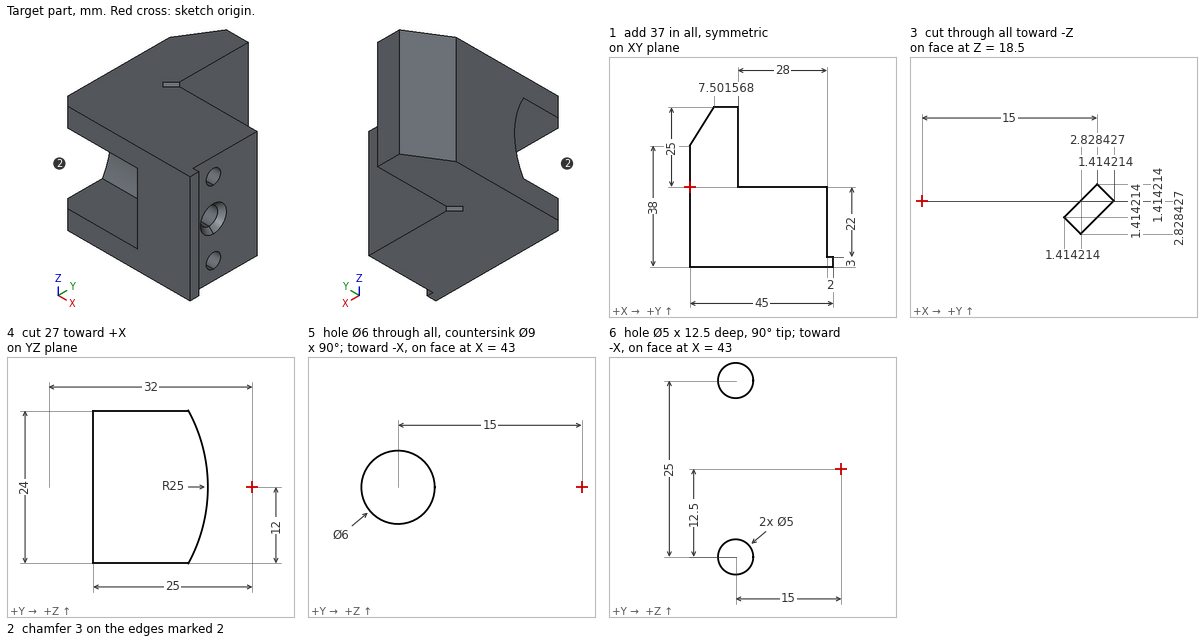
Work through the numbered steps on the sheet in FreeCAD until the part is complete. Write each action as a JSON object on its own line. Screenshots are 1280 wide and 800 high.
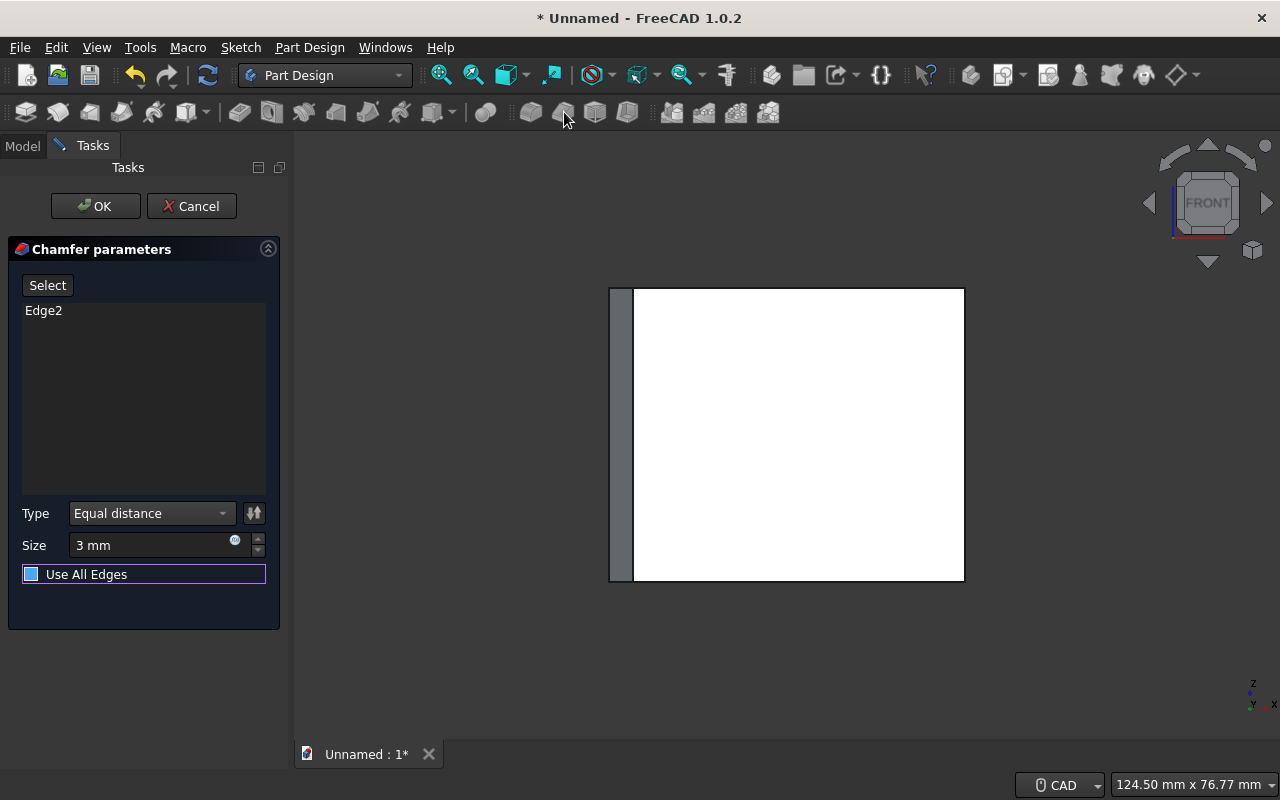
{"action": "left_click", "coordinate": [96, 206]}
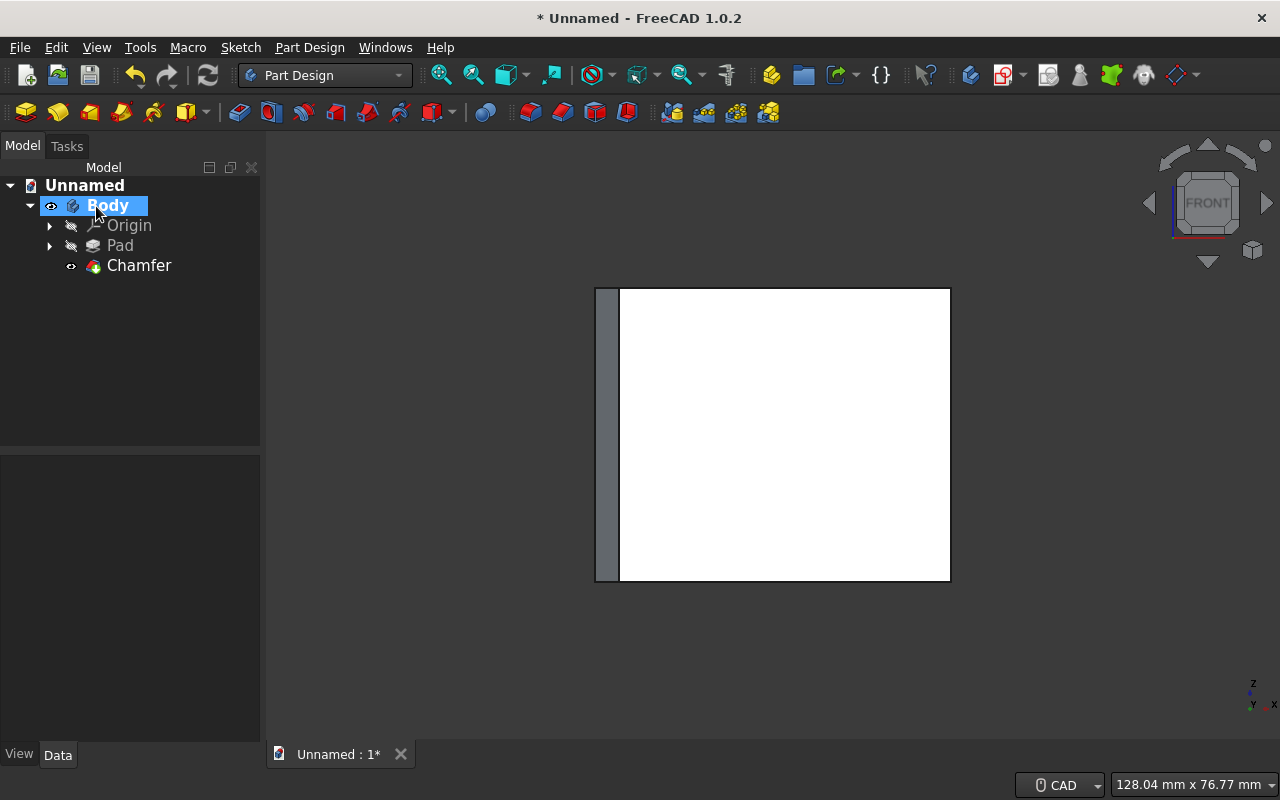
{"action": "key", "text": "0"}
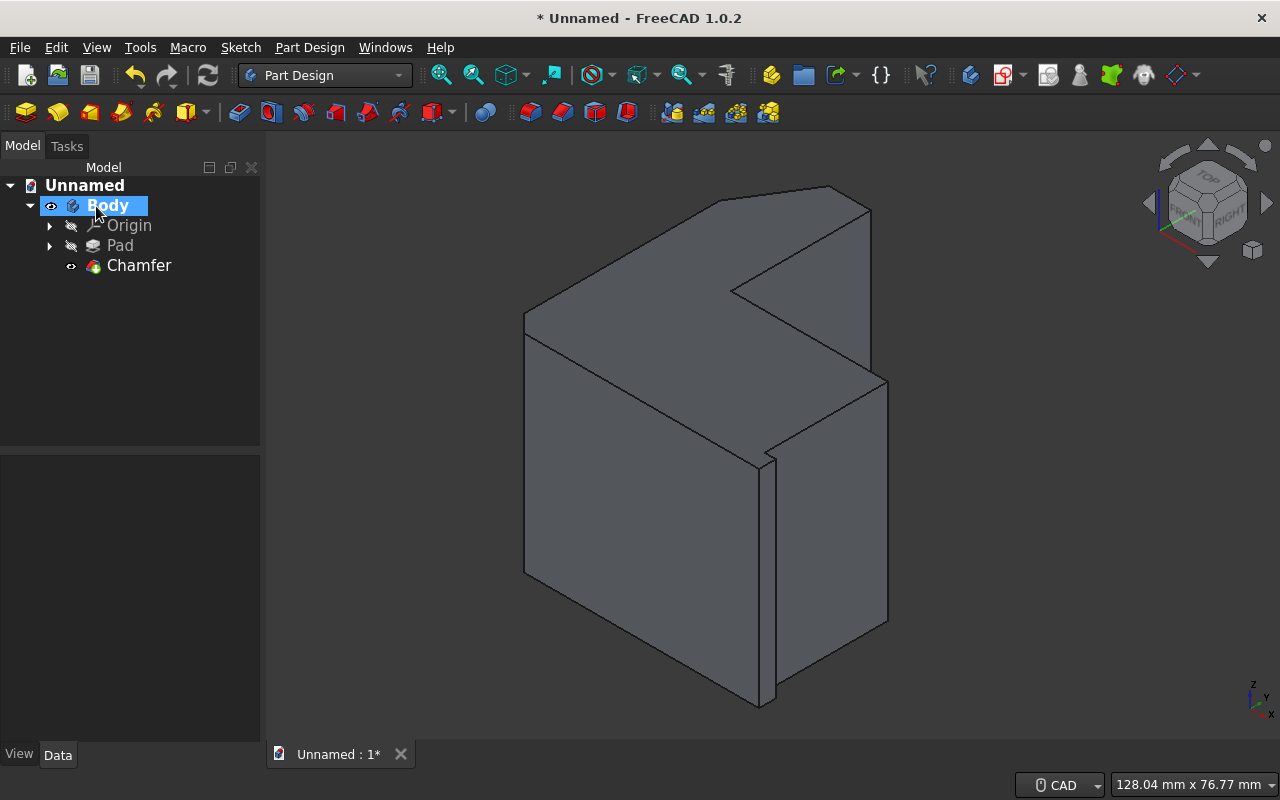
{"action": "left_click", "coordinate": [729, 381]}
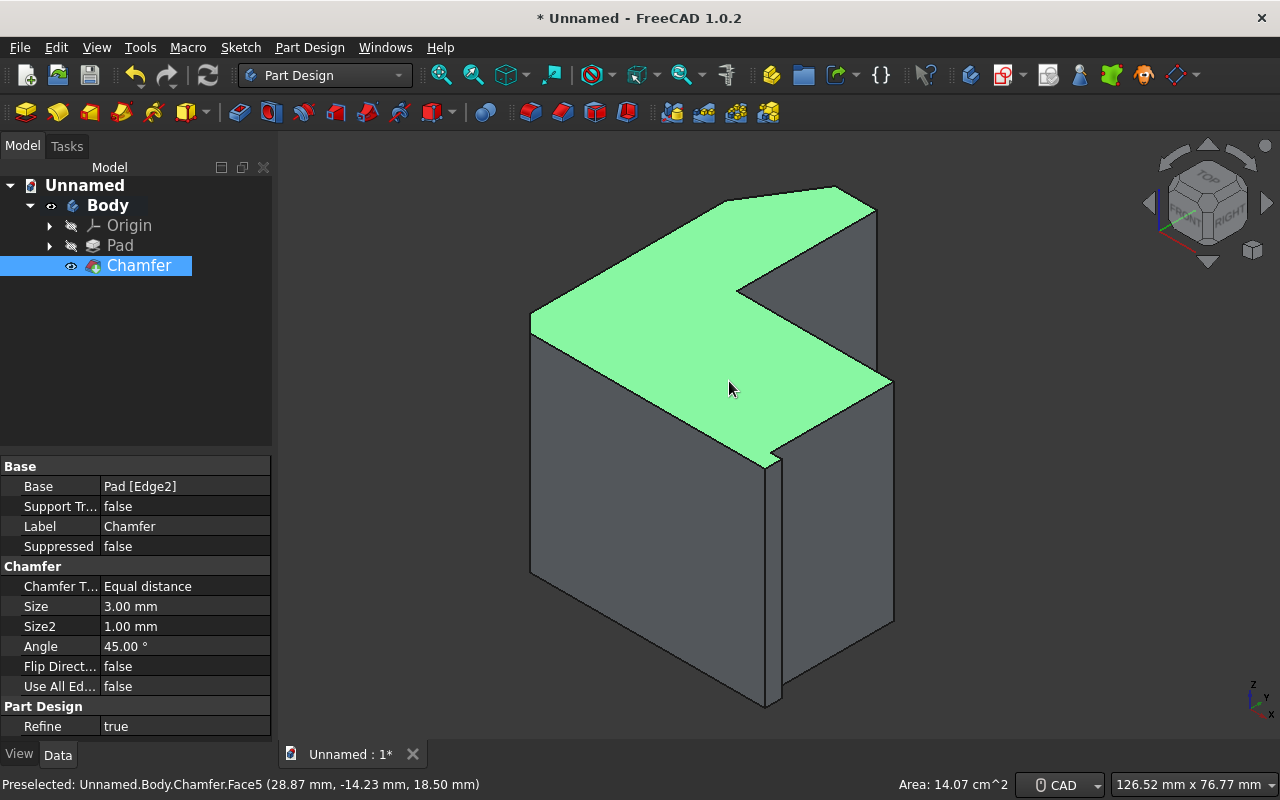
{"action": "left_click", "coordinate": [1004, 76]}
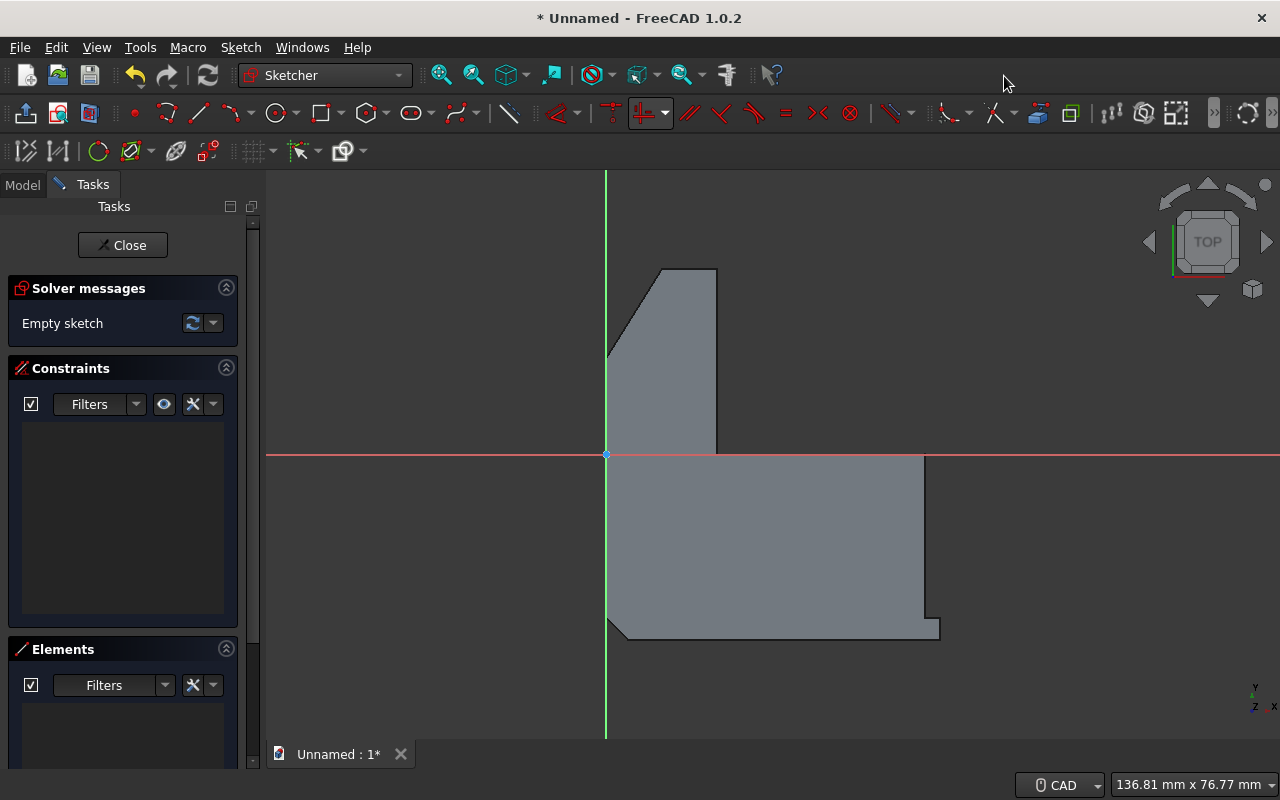
{"action": "scroll", "coordinate": [713, 460], "scroll_direction": "up", "scroll_amount": 12}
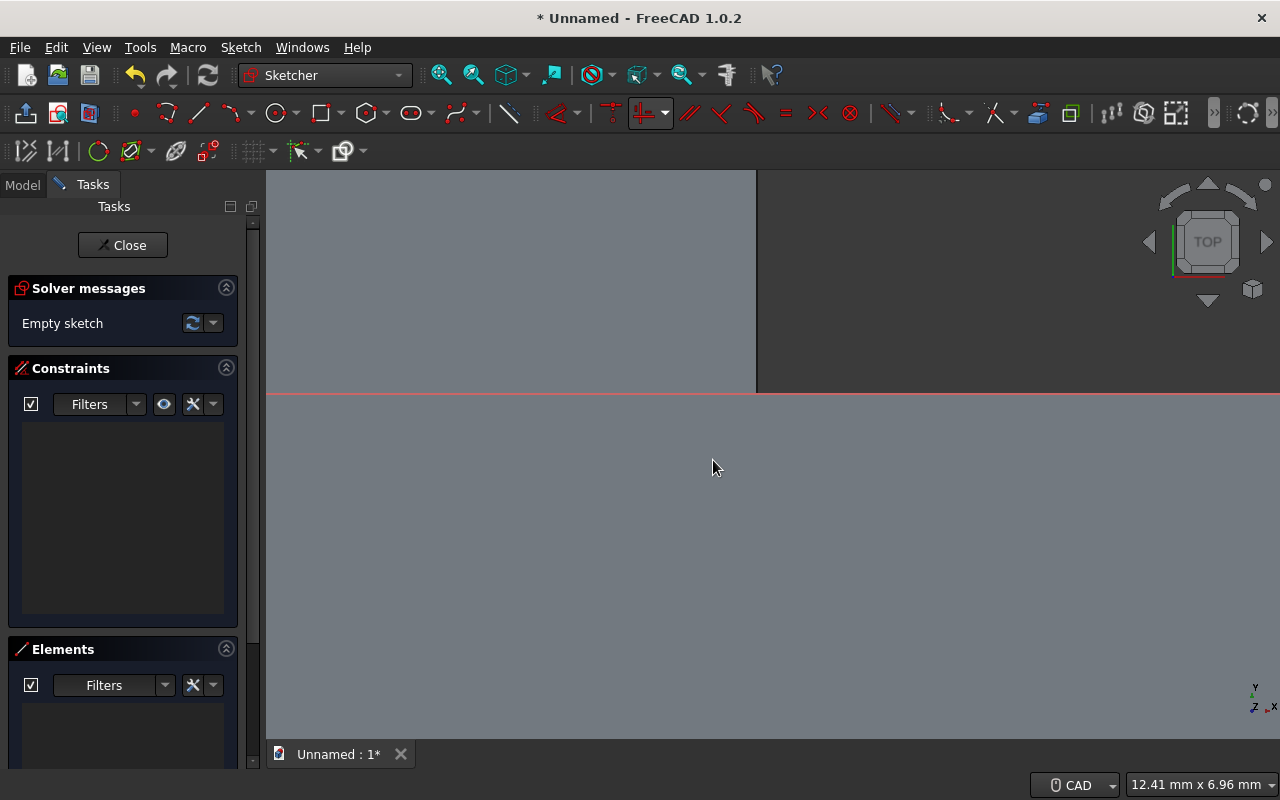
{"action": "left_click", "coordinate": [168, 114]}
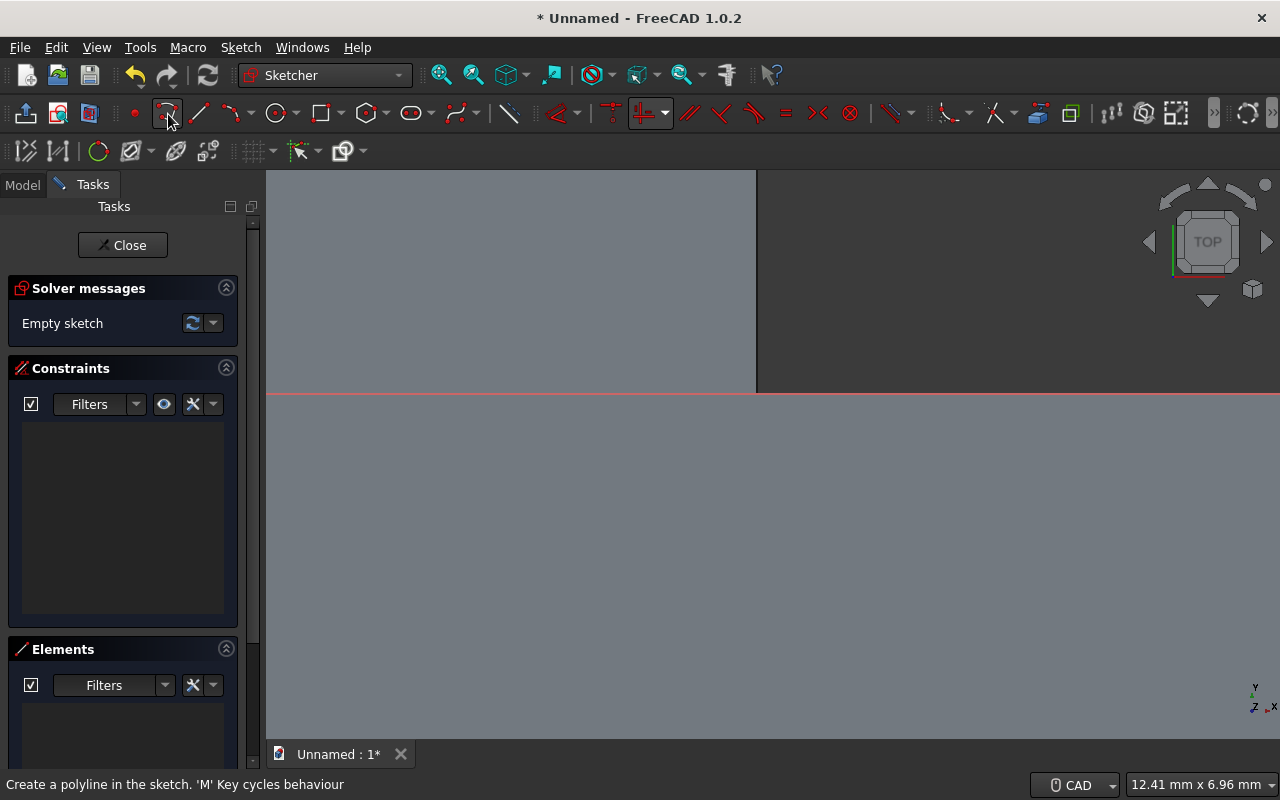
{"action": "left_click", "coordinate": [526, 510]}
{"action": "left_click", "coordinate": [642, 625]}
{"action": "left_click", "coordinate": [873, 394]}
{"action": "left_click", "coordinate": [757, 279]}
{"action": "left_click", "coordinate": [526, 511]}
{"action": "key", "text": "Escape"}
{"action": "key", "text": "Escape"}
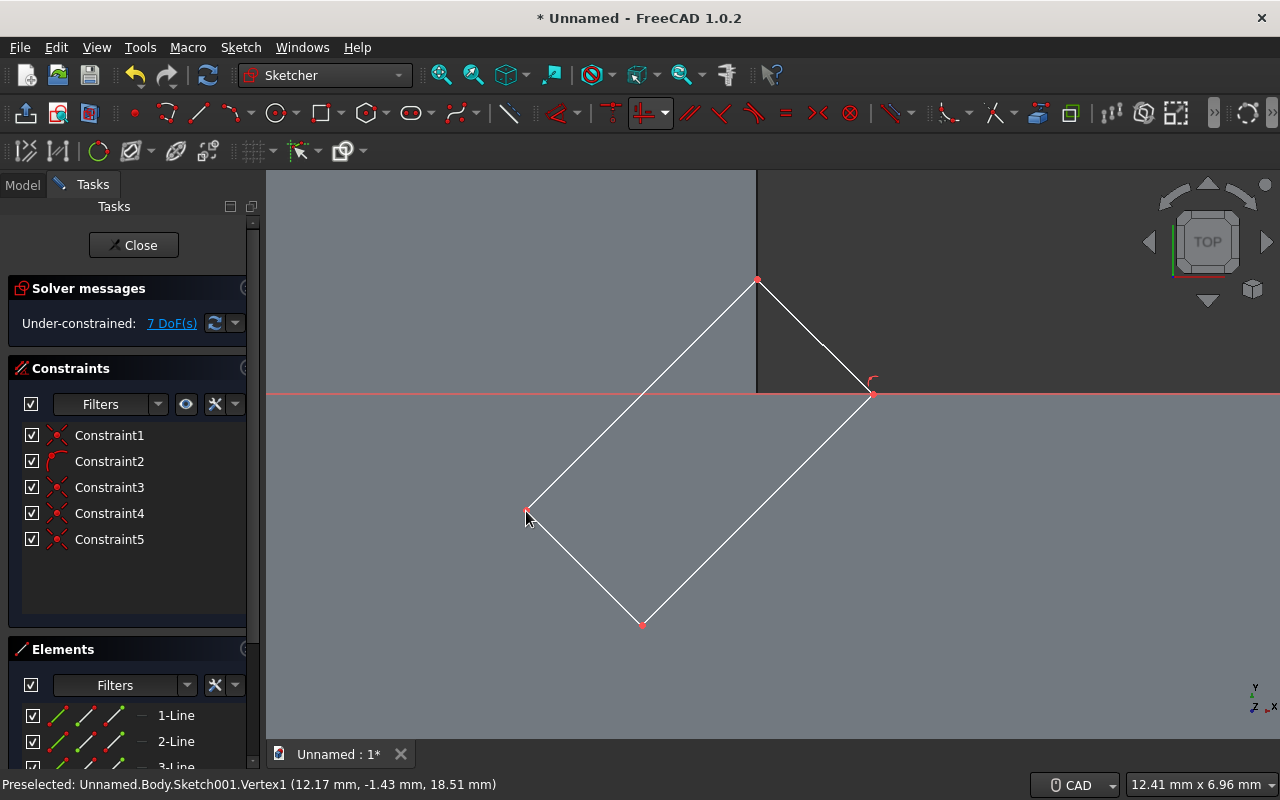
{"action": "left_click", "coordinate": [556, 114]}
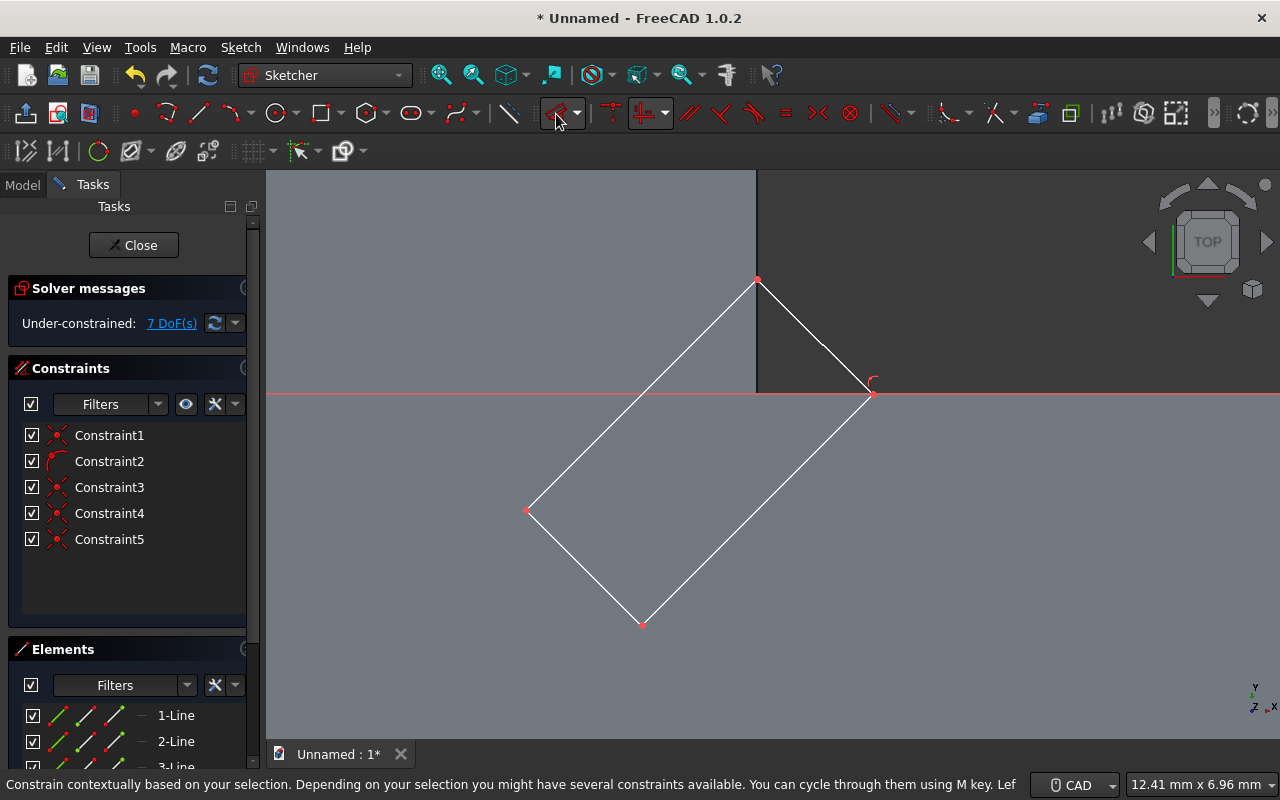
{"action": "left_click", "coordinate": [757, 280]}
{"action": "left_click", "coordinate": [526, 246]}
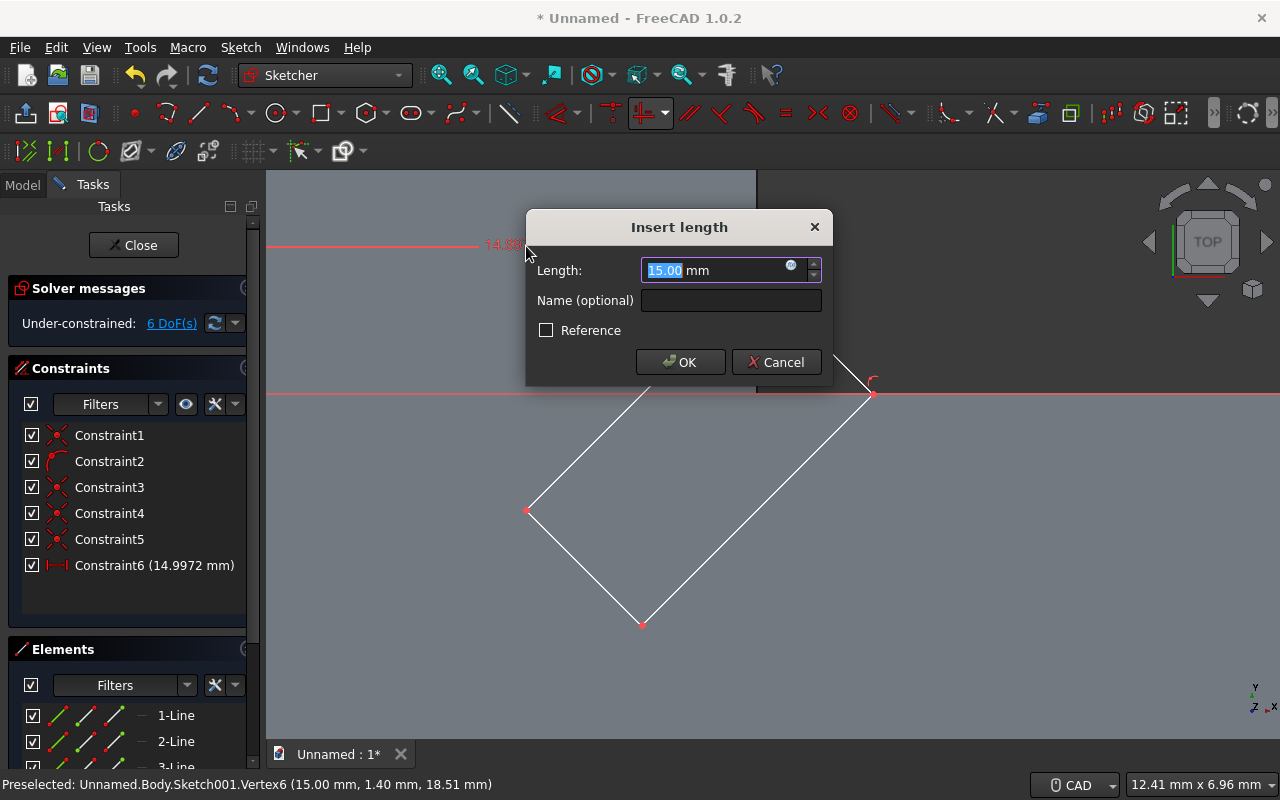
{"action": "type", "text": "15"}
{"action": "key", "text": "Return"}